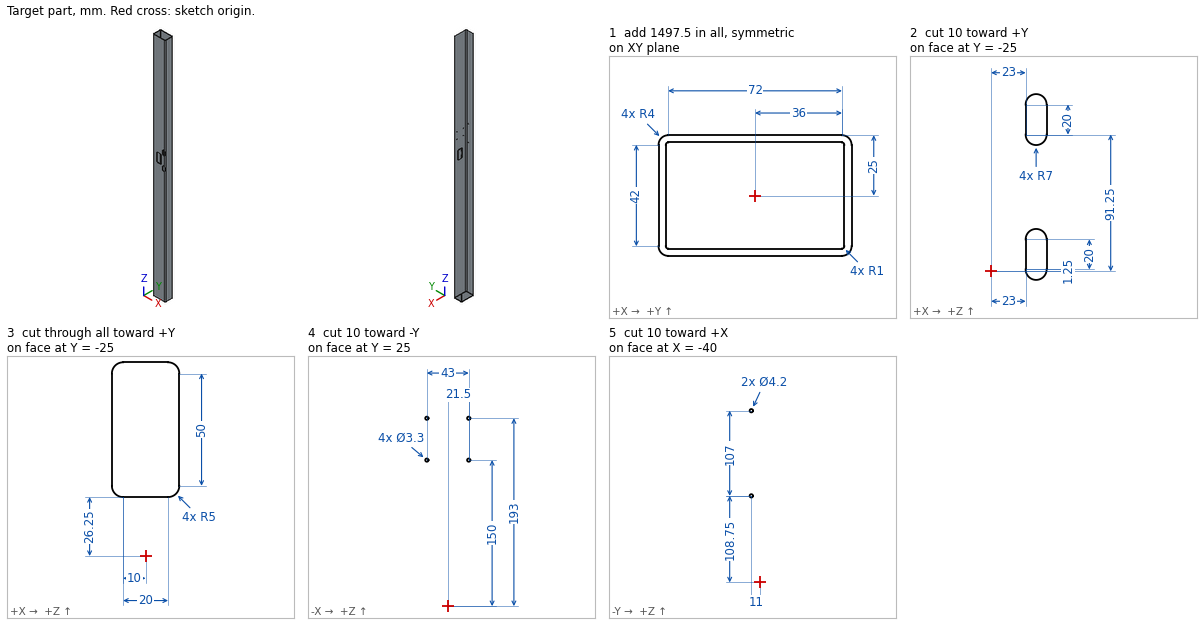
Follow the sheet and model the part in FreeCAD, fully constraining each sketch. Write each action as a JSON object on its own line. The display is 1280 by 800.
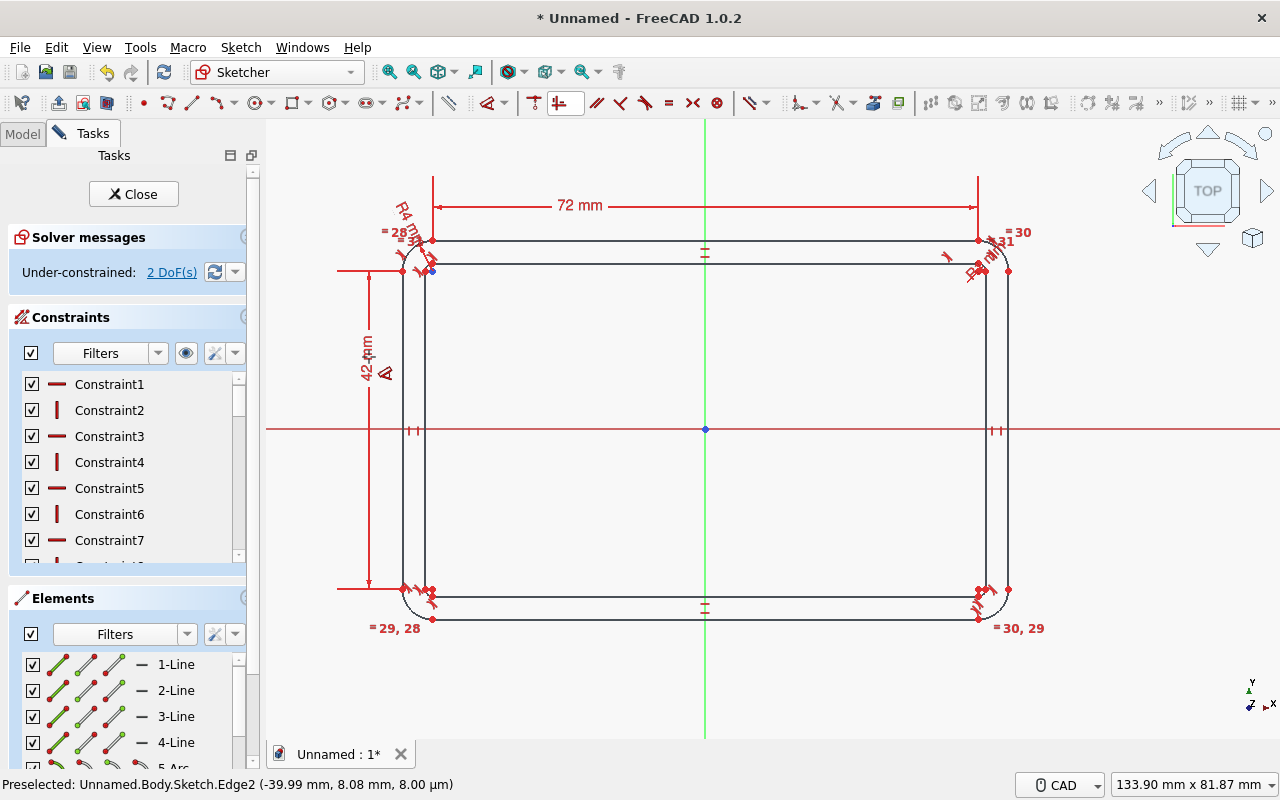
{"action": "left_click", "coordinate": [978, 241]}
{"action": "left_click", "coordinate": [842, 207]}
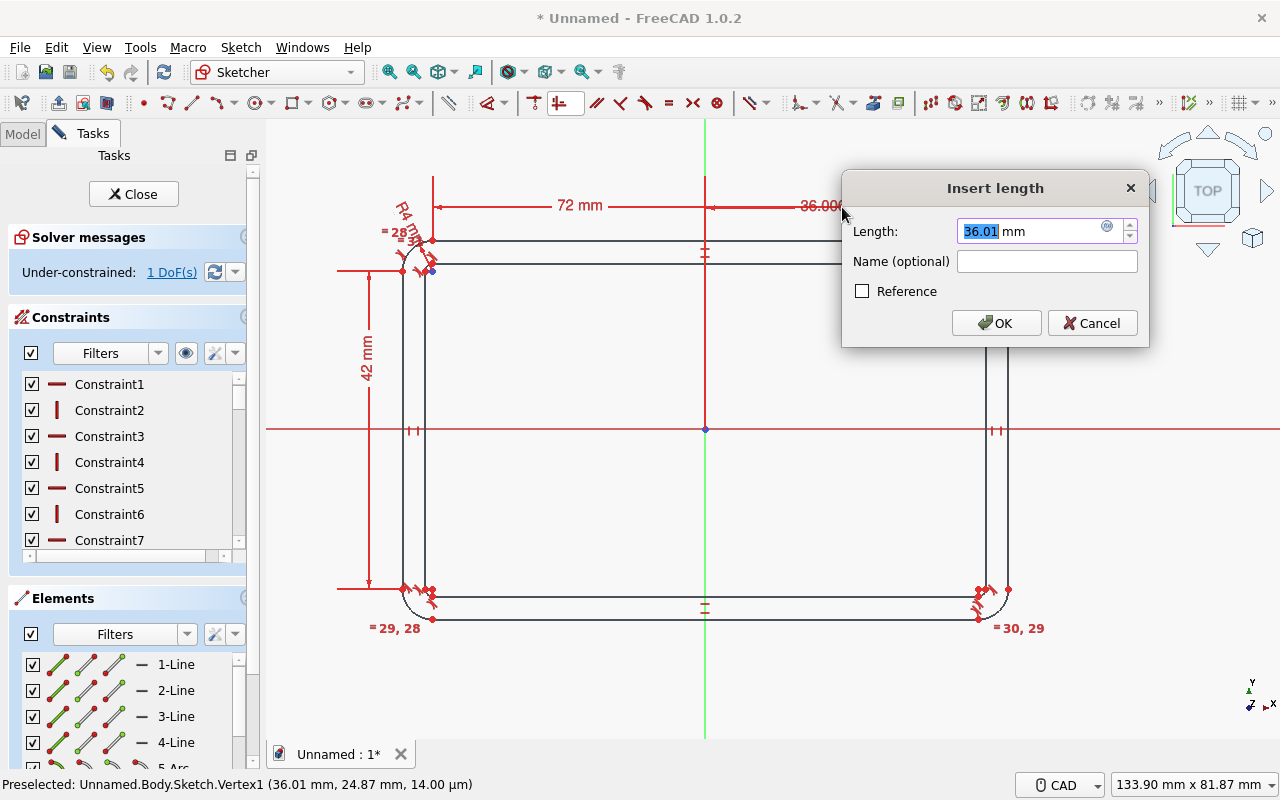
{"action": "type", "text": "36"}
{"action": "key", "text": "Return"}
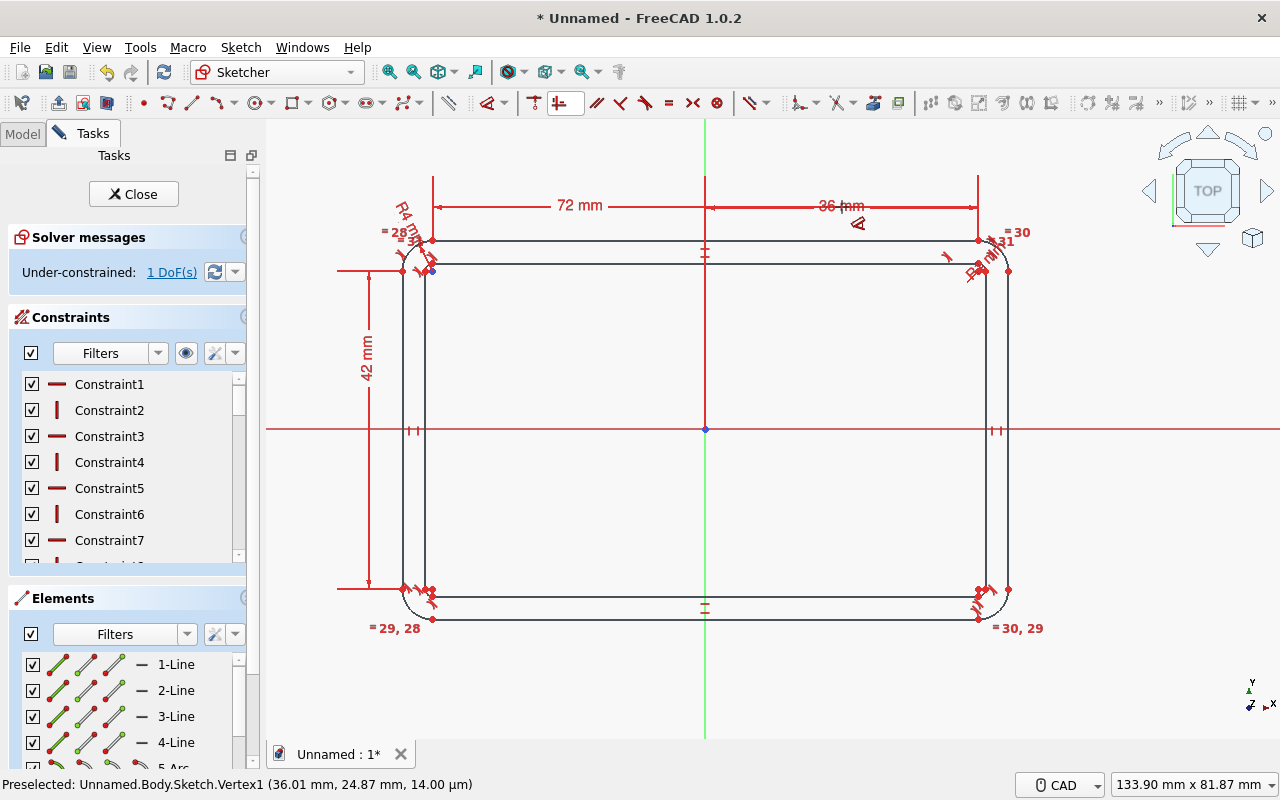
{"action": "left_click", "coordinate": [978, 241]}
{"action": "left_click", "coordinate": [671, 335]}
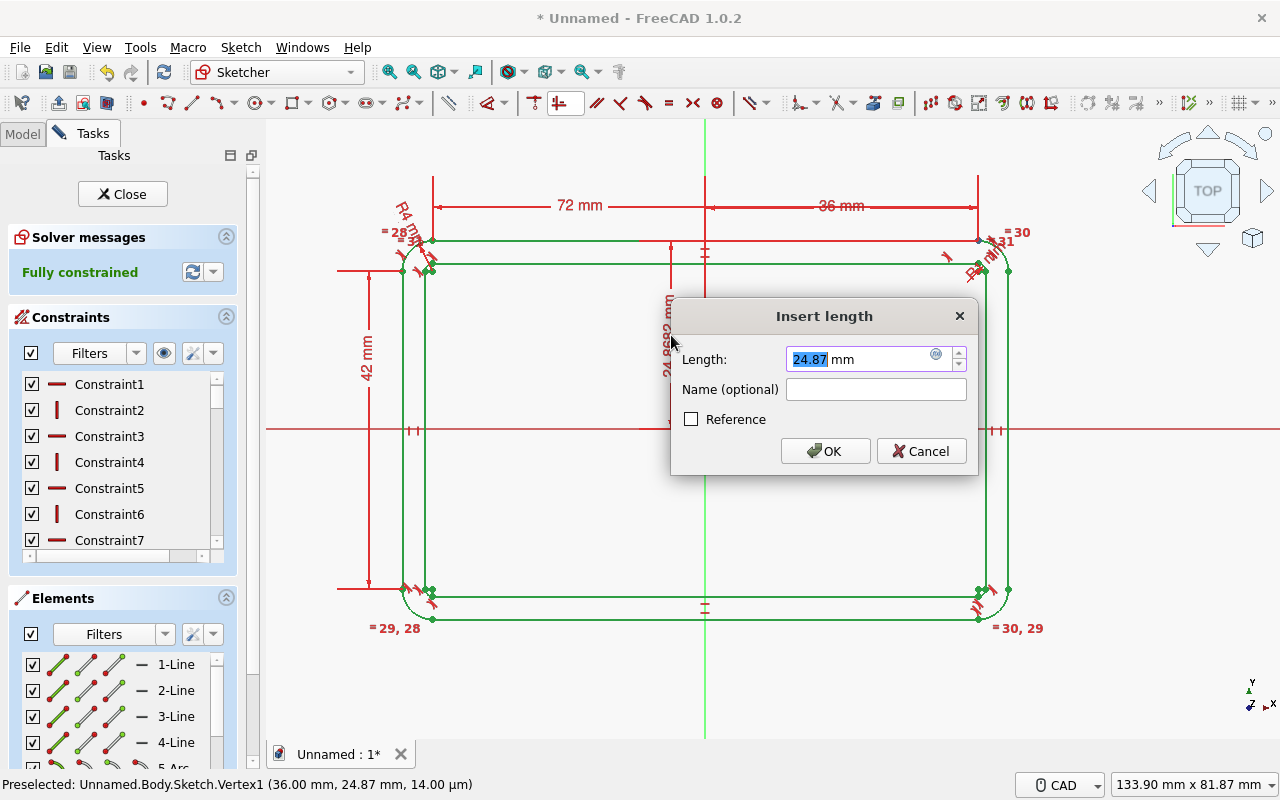
{"action": "type", "text": "25"}
{"action": "key", "text": "Return"}
{"action": "key", "text": "Escape"}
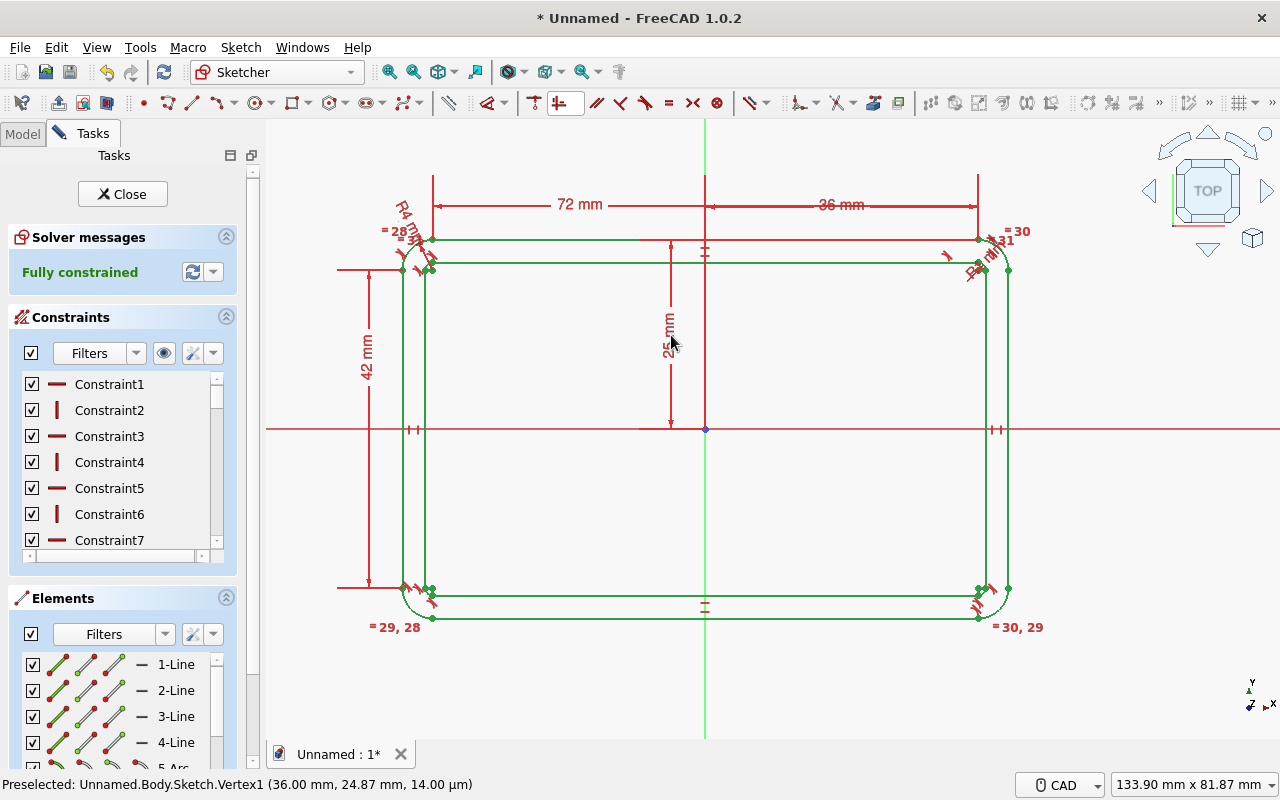
{"action": "left_click", "coordinate": [123, 194]}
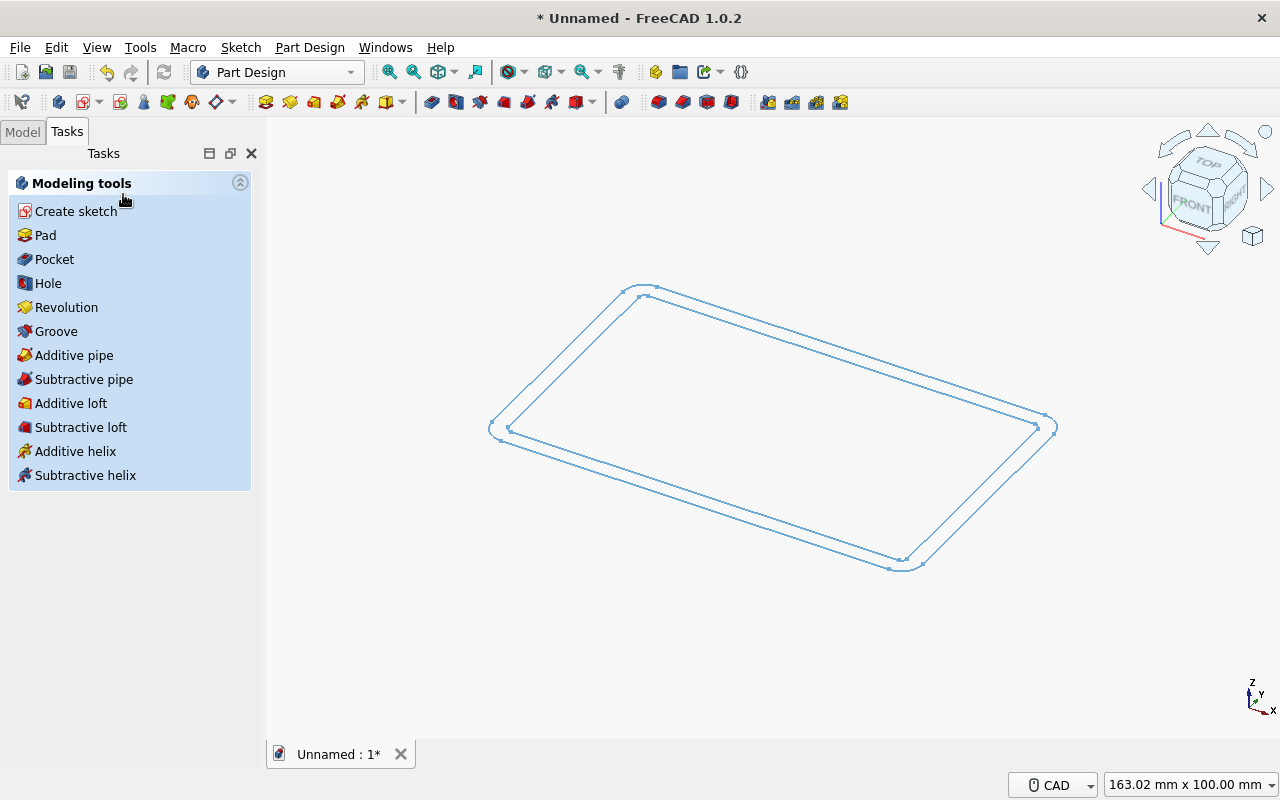
{"action": "left_click", "coordinate": [266, 102]}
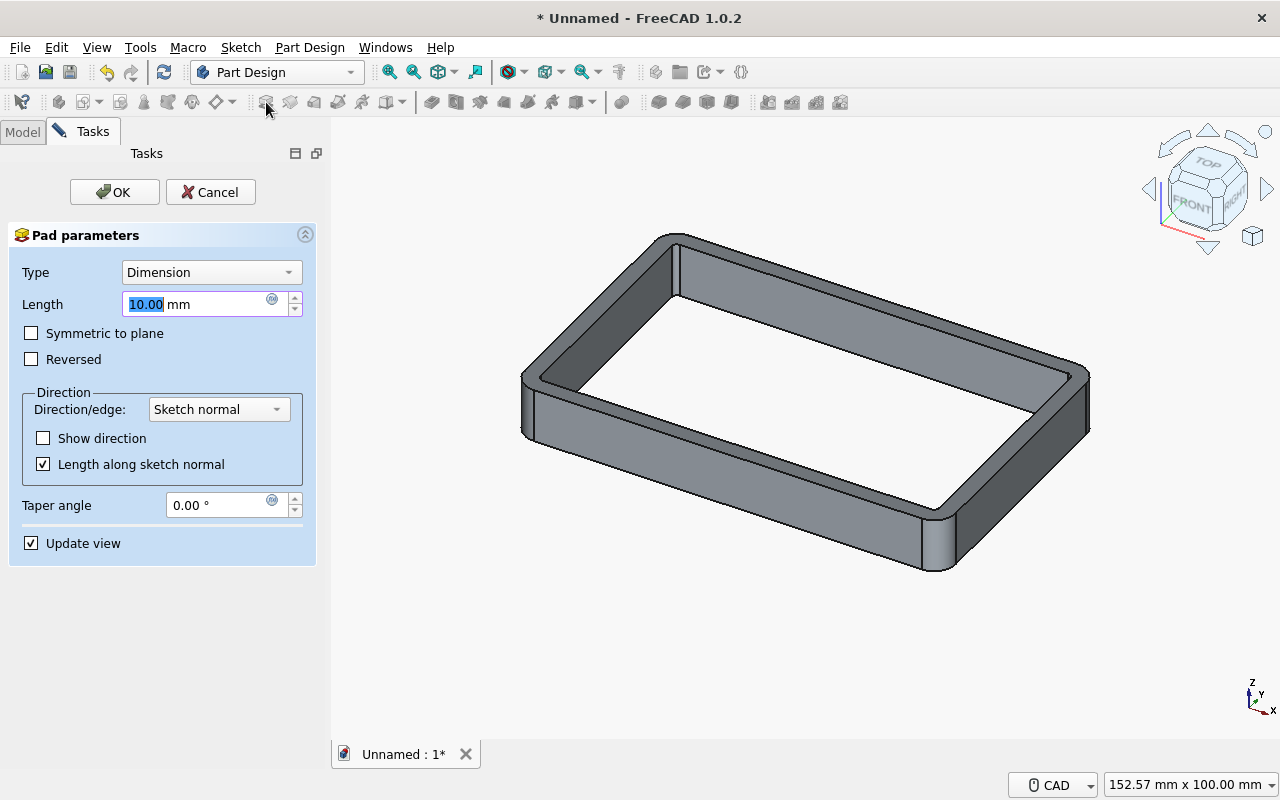
{"action": "type", "text": "1497.5"}
{"action": "key", "text": "Tab"}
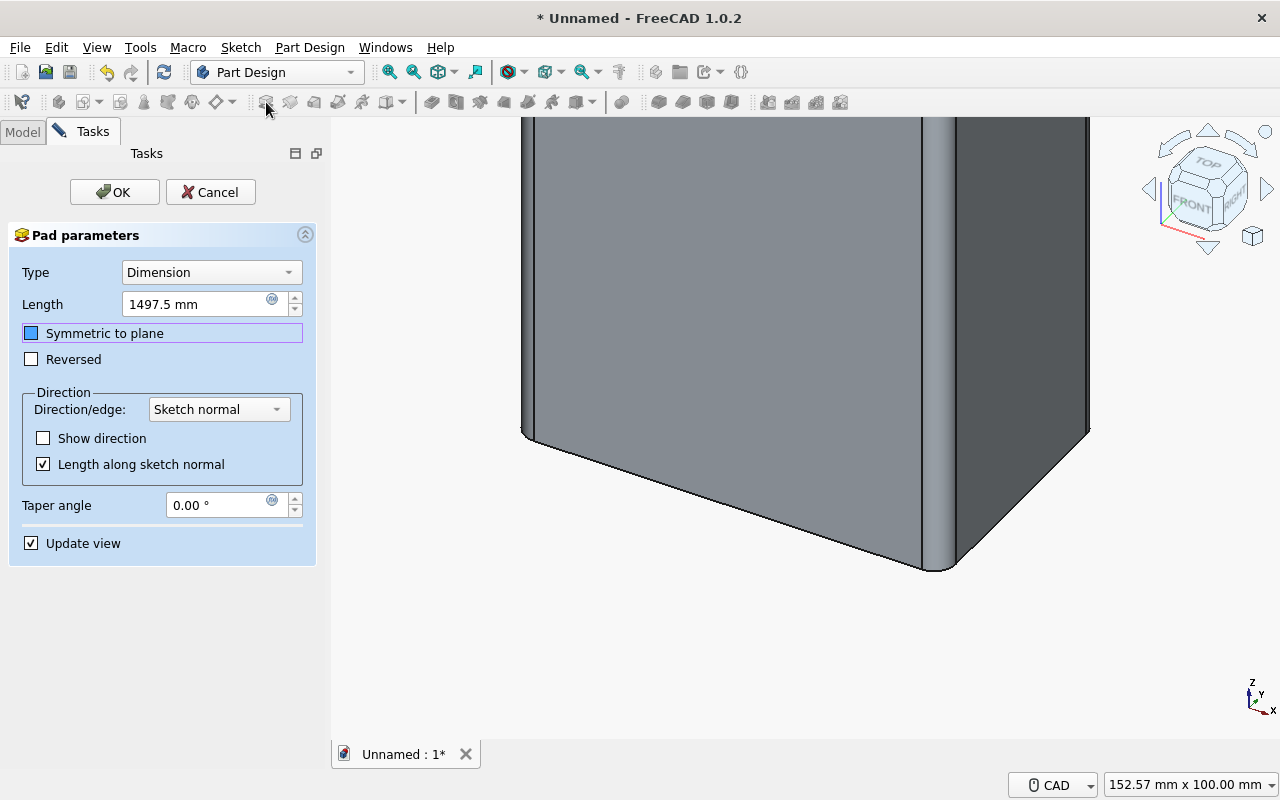
{"action": "left_click", "coordinate": [30, 333]}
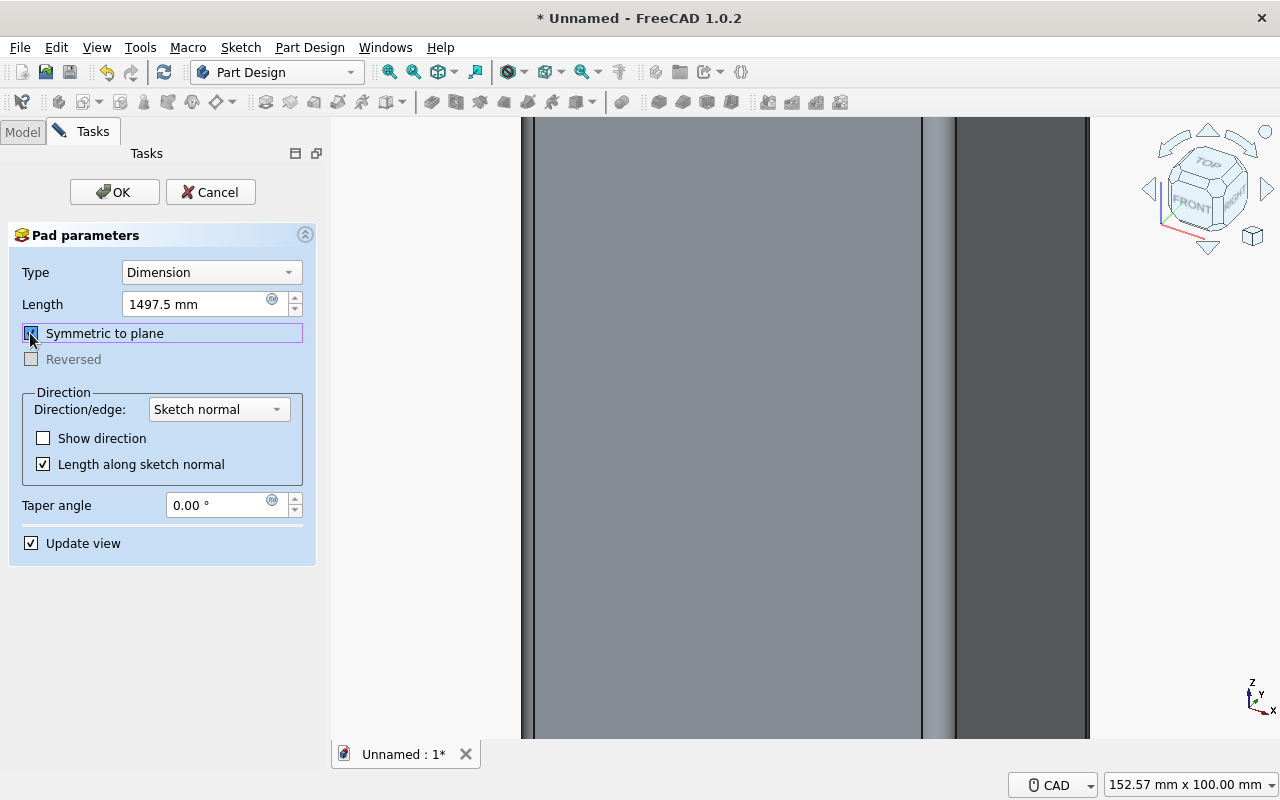
{"action": "left_click", "coordinate": [115, 192]}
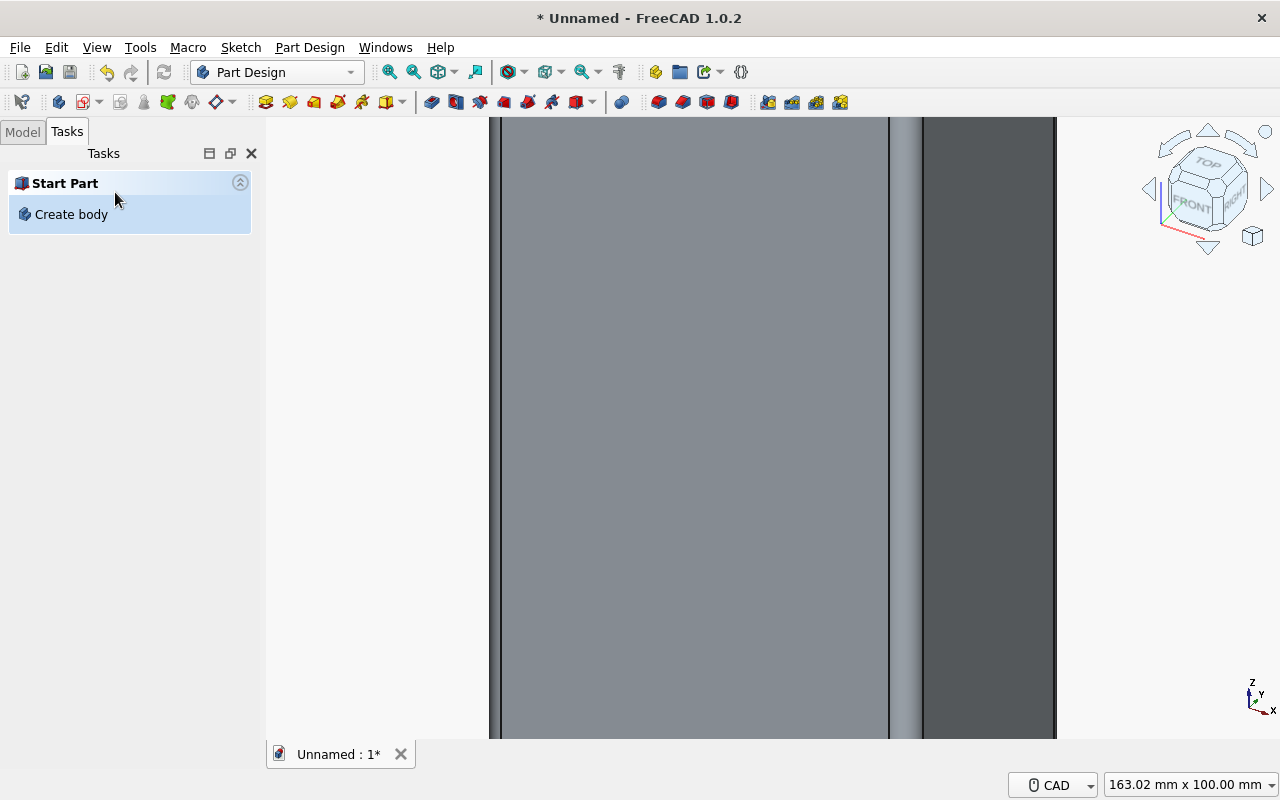
{"action": "key", "text": "v f"}